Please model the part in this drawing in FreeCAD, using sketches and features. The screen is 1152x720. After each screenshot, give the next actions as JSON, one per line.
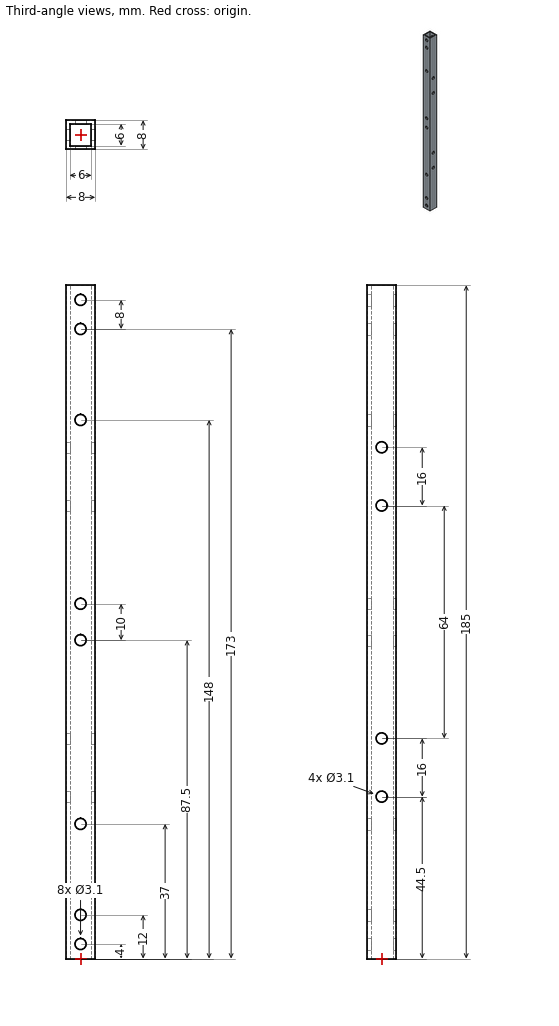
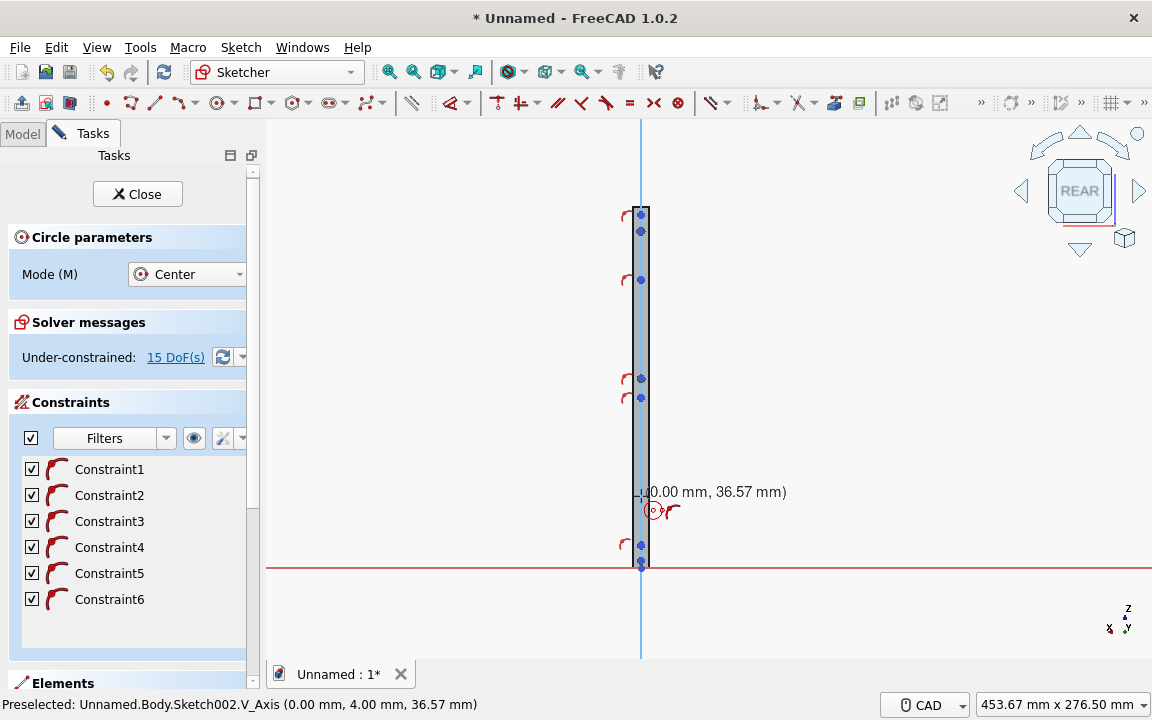
{"action": "left_click", "coordinate": [641, 496]}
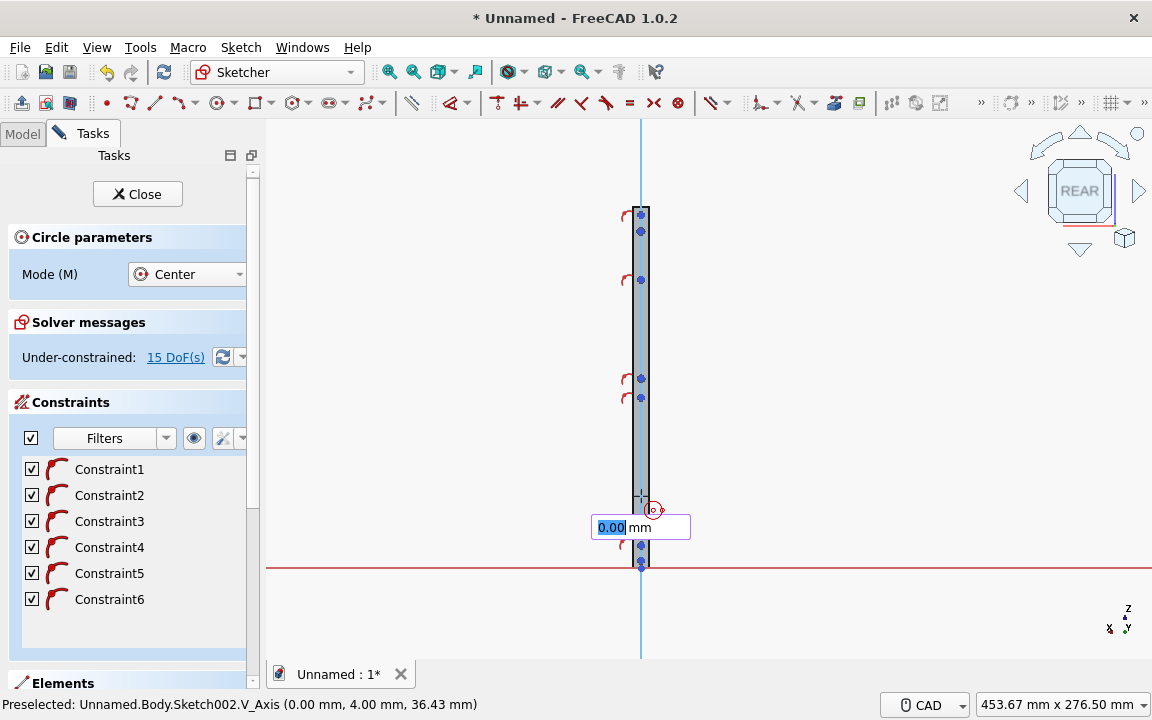
{"action": "scroll", "coordinate": [644, 495], "scroll_direction": "up", "scroll_amount": 9}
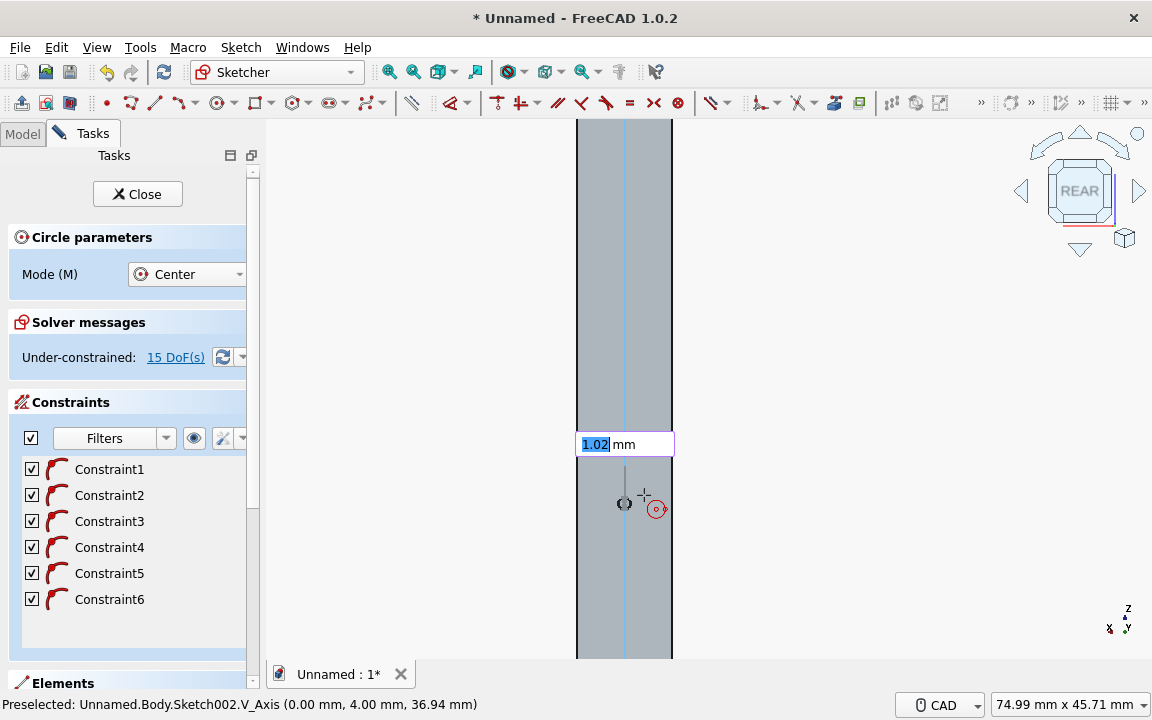
{"action": "left_click", "coordinate": [642, 491]}
{"action": "key", "text": "Escape"}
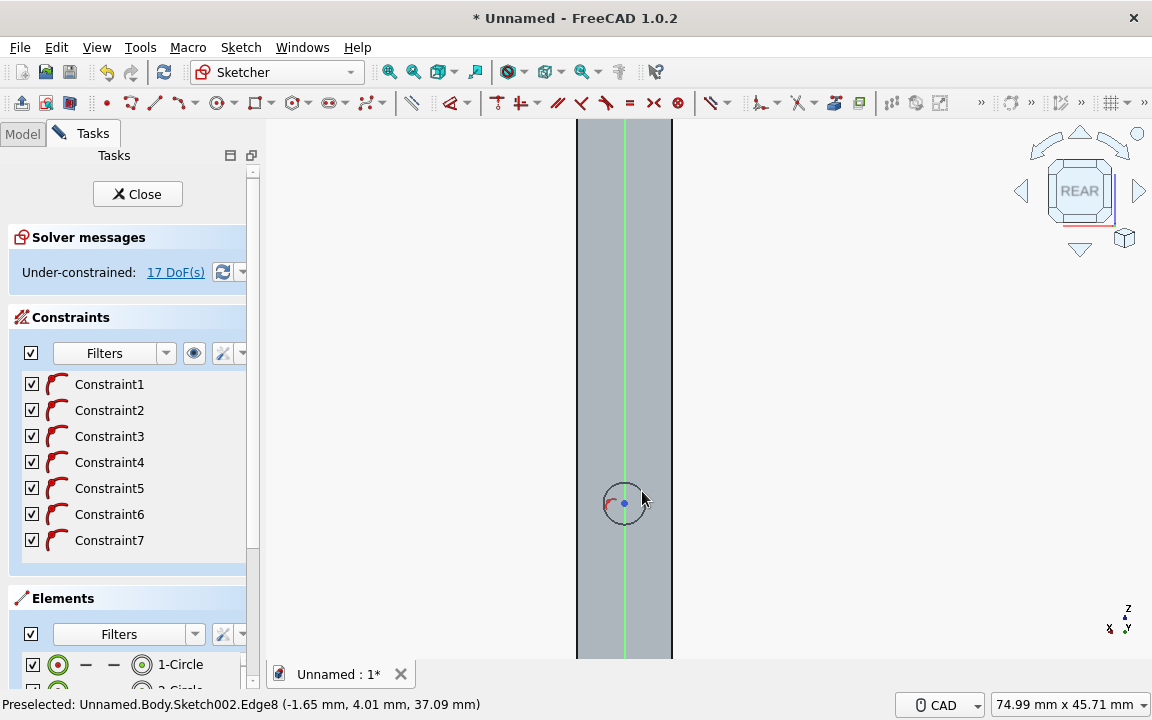
{"action": "scroll", "coordinate": [644, 495], "scroll_direction": "down", "scroll_amount": 9}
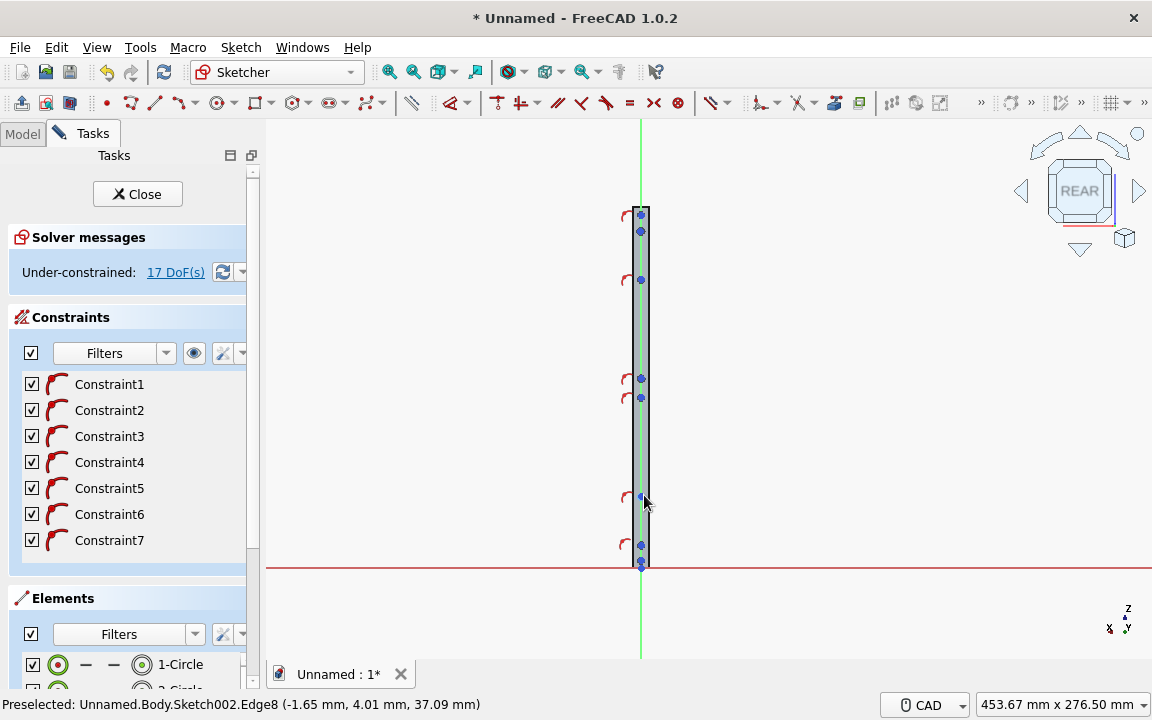
{"action": "scroll", "coordinate": [643, 558], "scroll_direction": "up", "scroll_amount": 10}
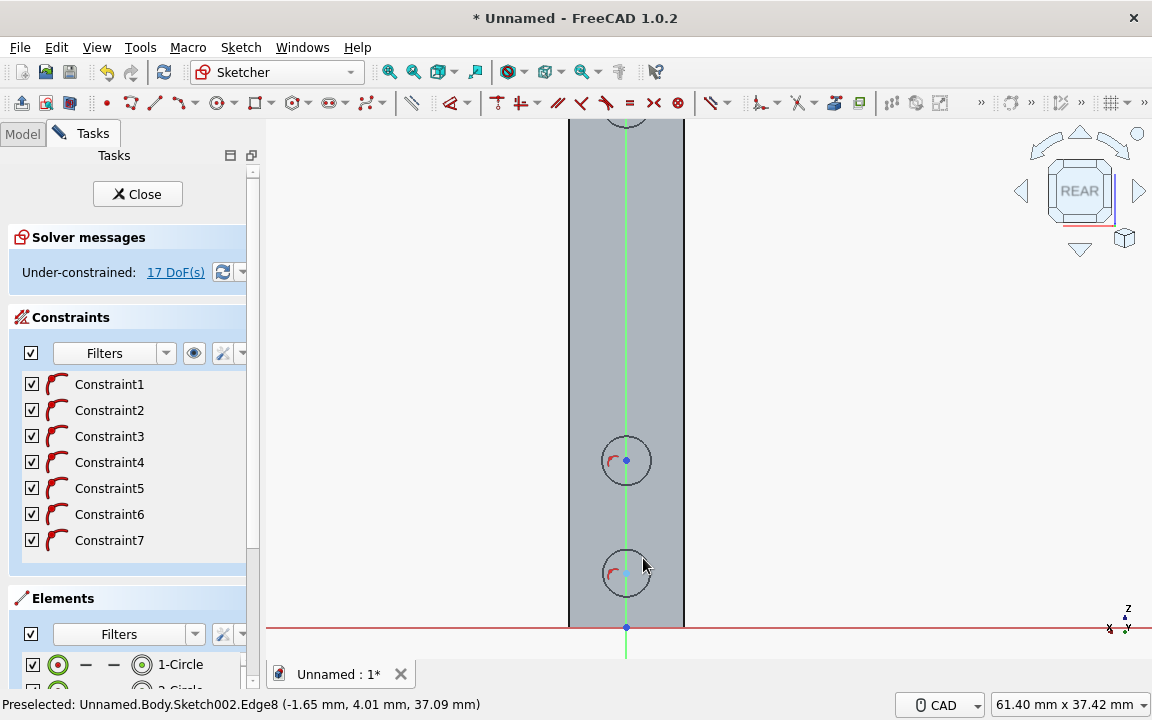
{"action": "left_click", "coordinate": [643, 556]}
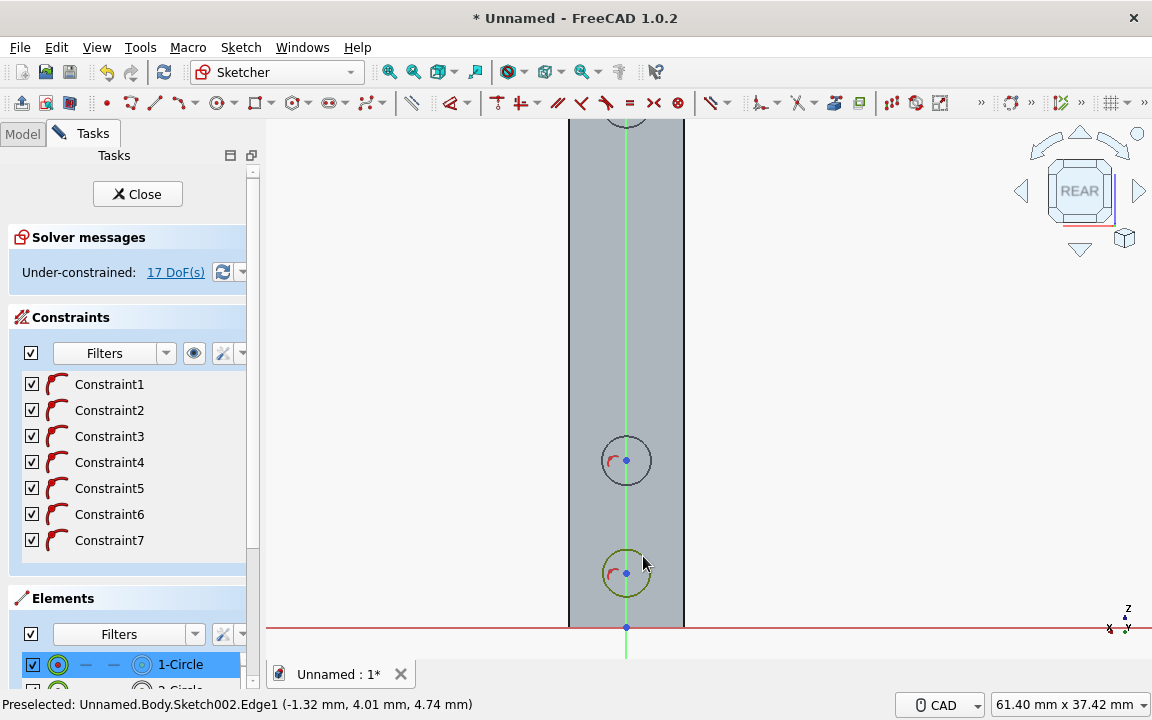
{"action": "left_click", "coordinate": [644, 443]}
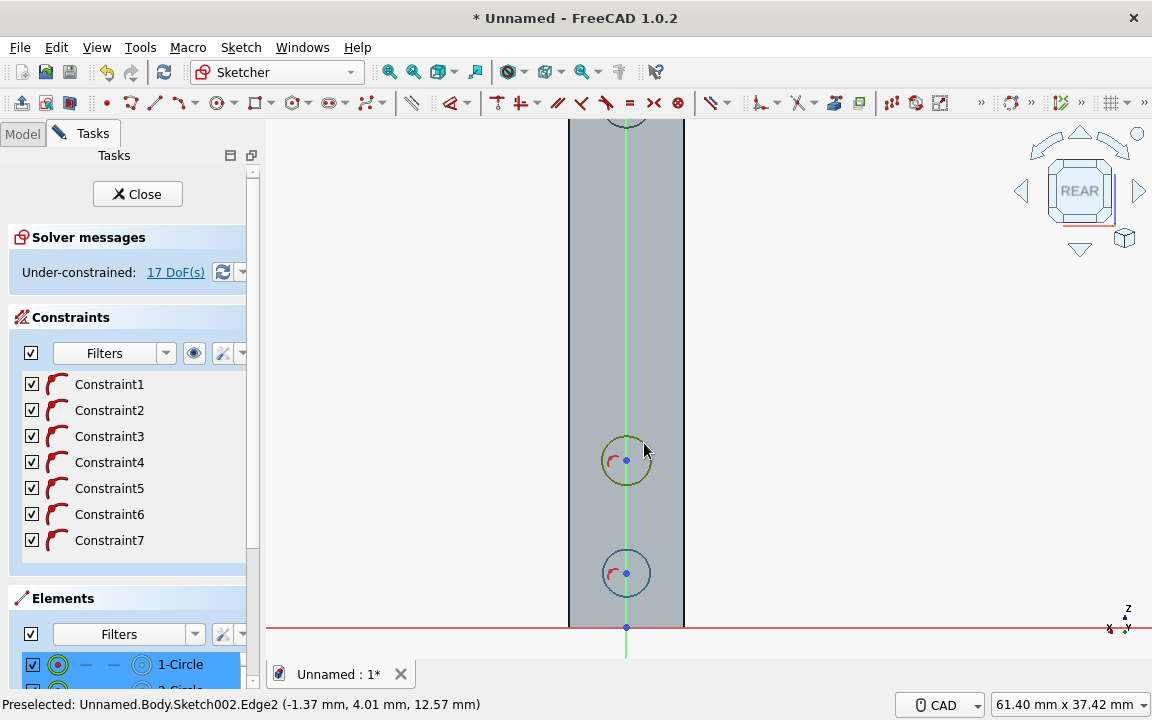
{"action": "scroll", "coordinate": [643, 558], "scroll_direction": "down", "scroll_amount": 10}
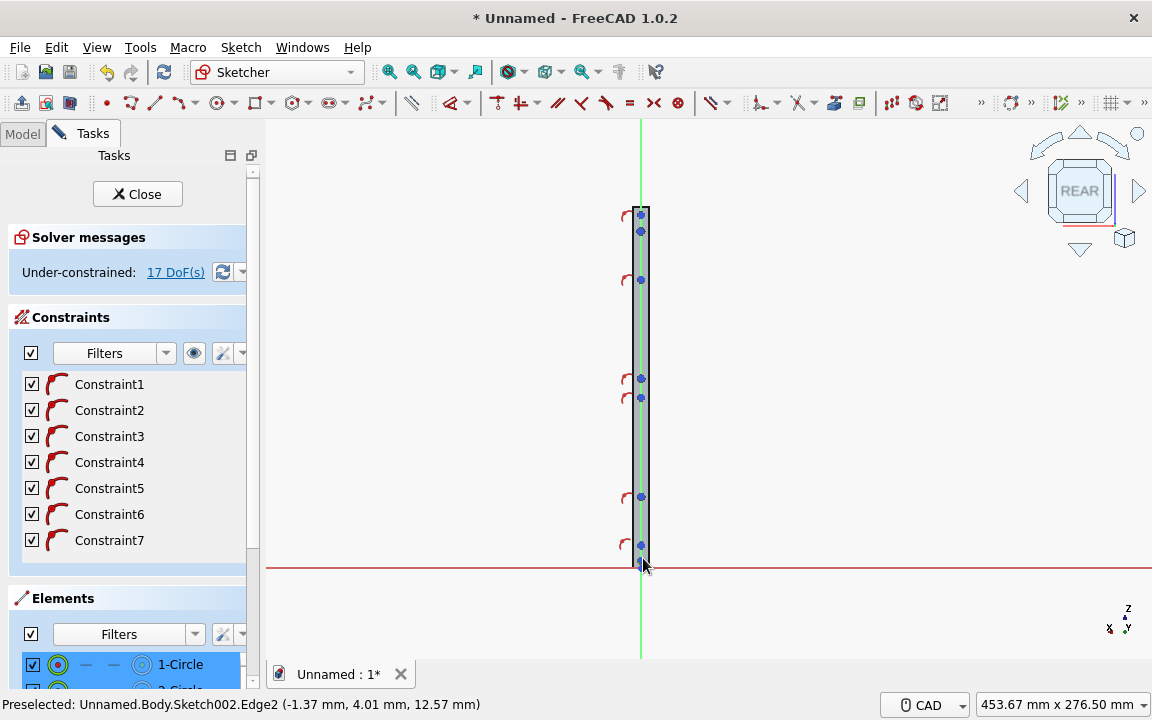
{"action": "scroll", "coordinate": [643, 229], "scroll_direction": "up", "scroll_amount": 9}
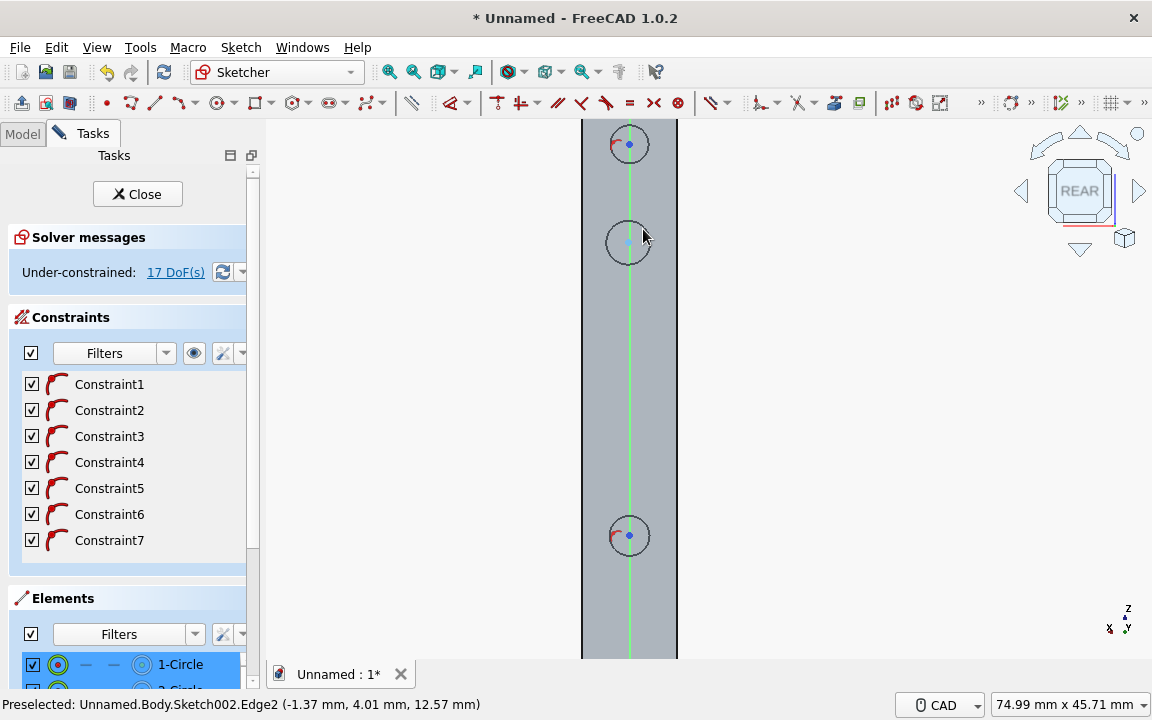
{"action": "left_click", "coordinate": [644, 227]}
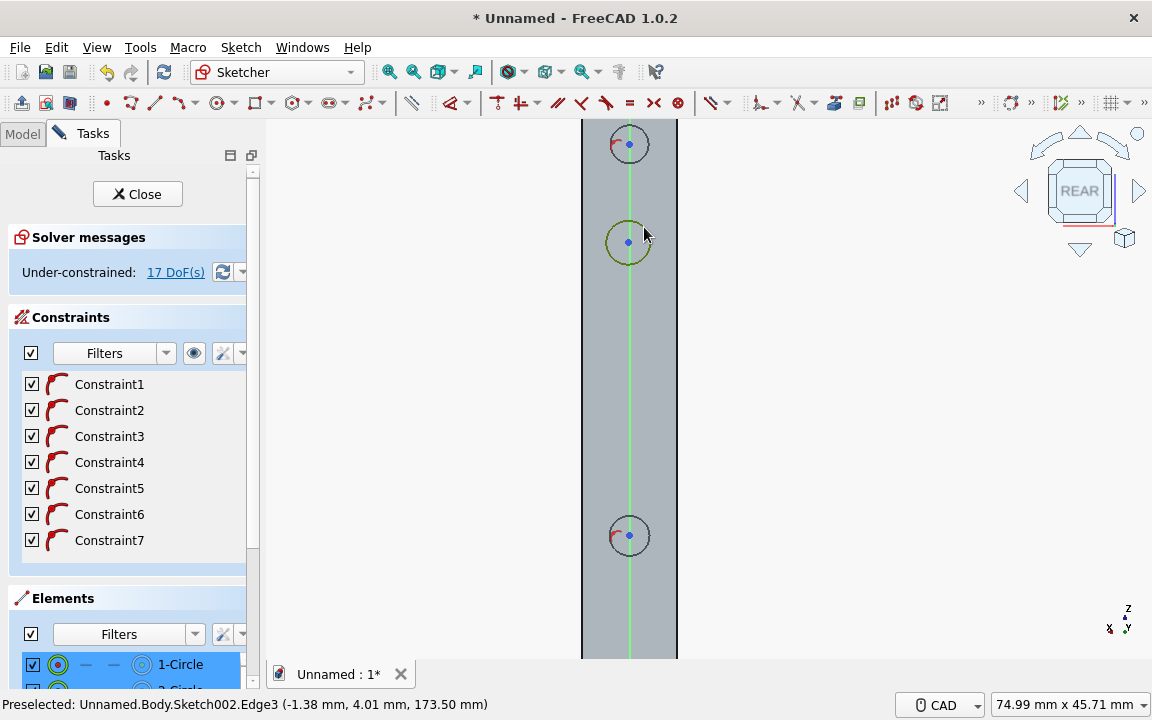
{"action": "left_click", "coordinate": [616, 158]}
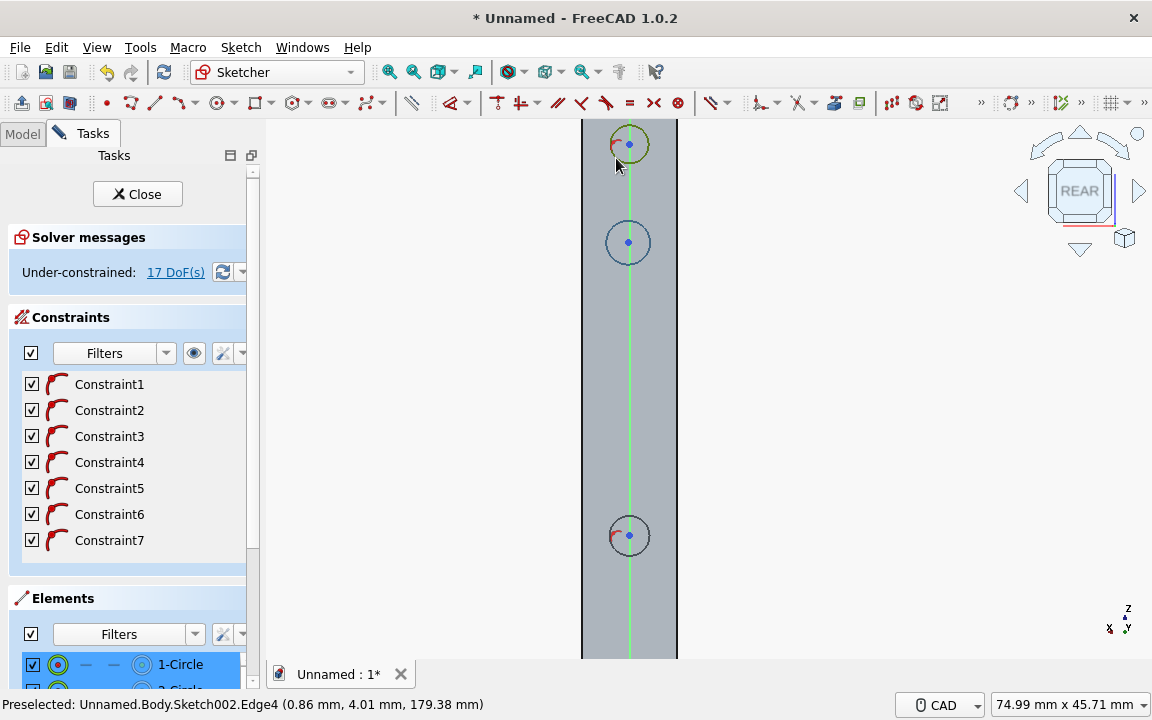
{"action": "scroll", "coordinate": [643, 228], "scroll_direction": "down", "scroll_amount": 9}